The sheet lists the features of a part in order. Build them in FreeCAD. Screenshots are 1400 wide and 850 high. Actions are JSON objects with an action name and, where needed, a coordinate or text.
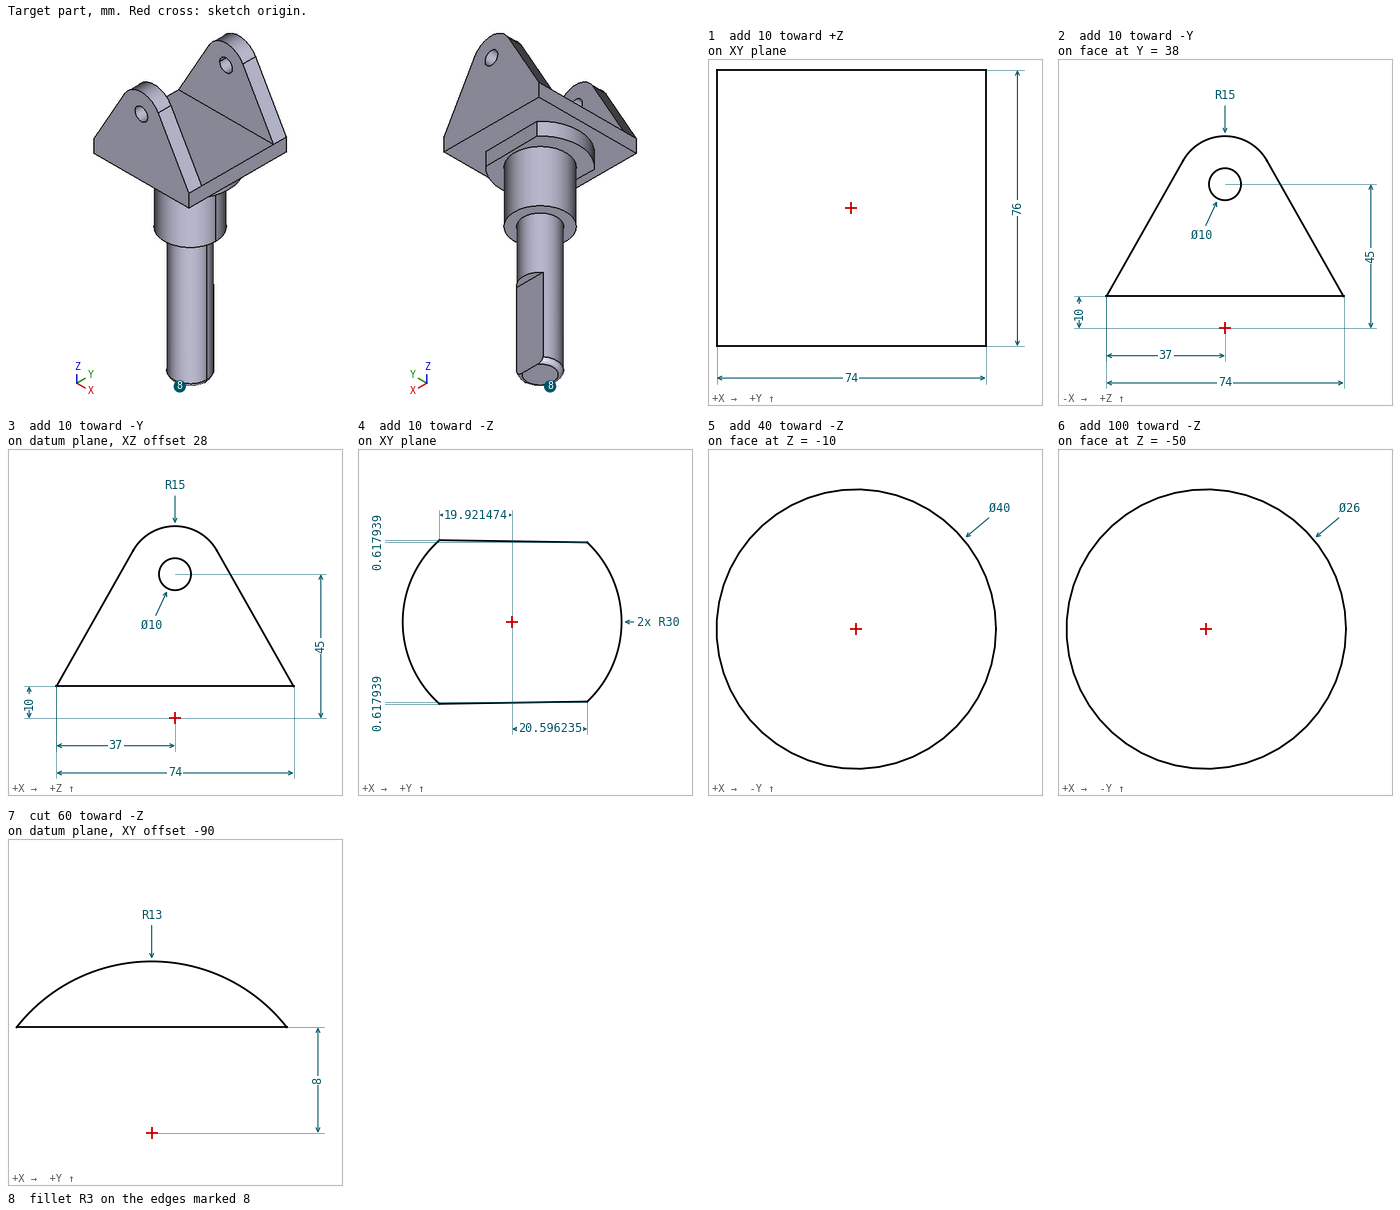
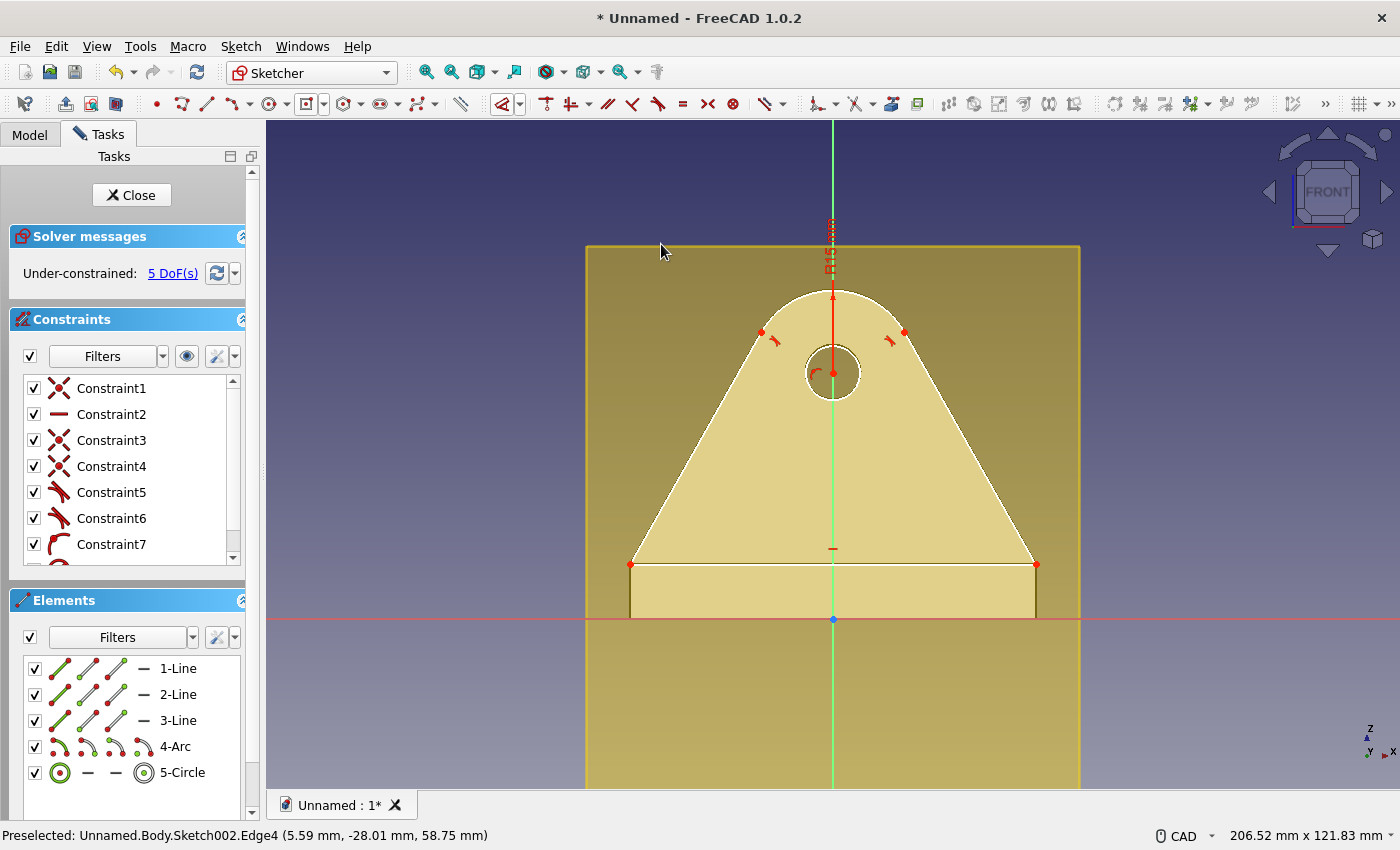
{"action": "left_click", "coordinate": [852, 354]}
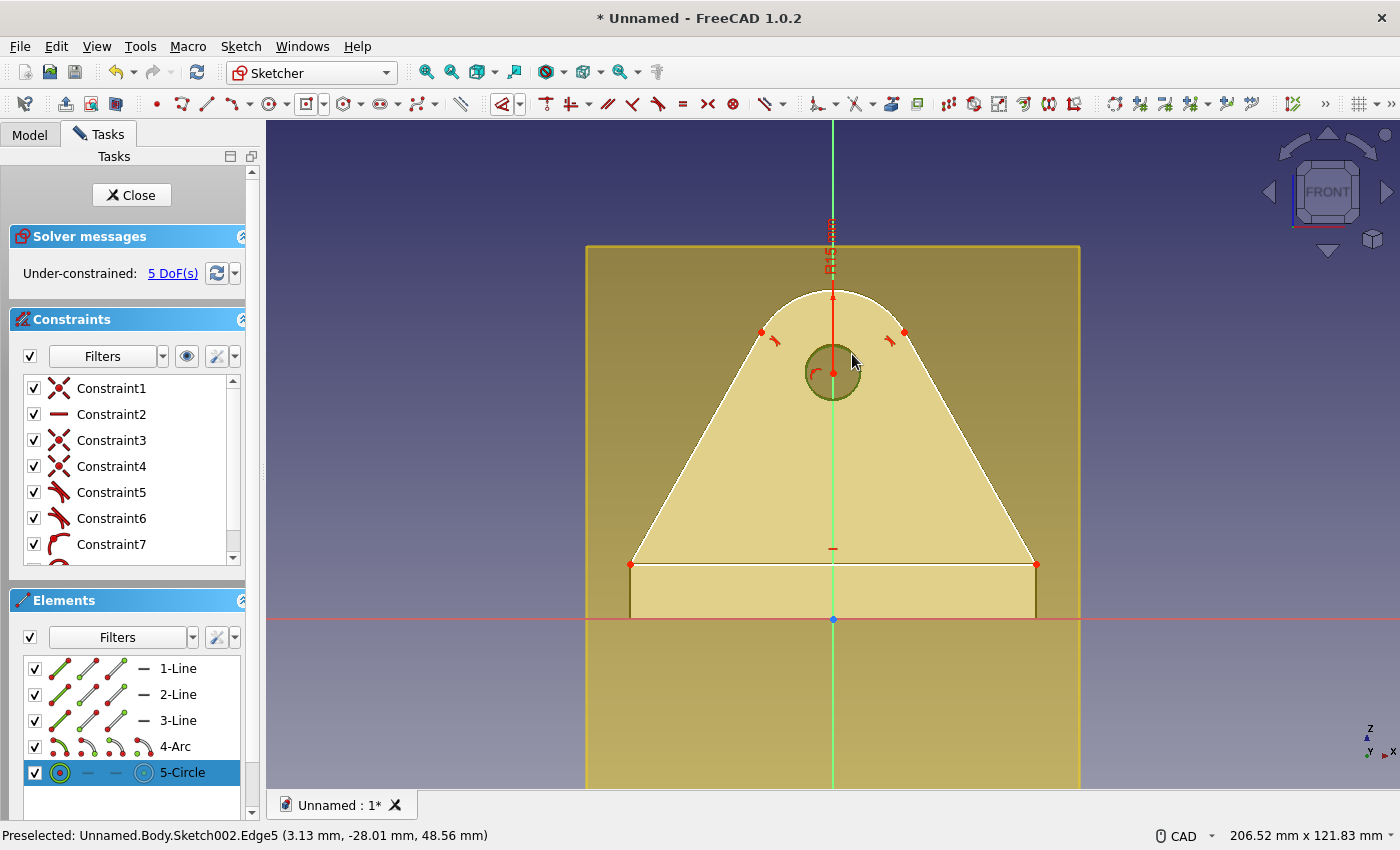
{"action": "key", "text": "k o"}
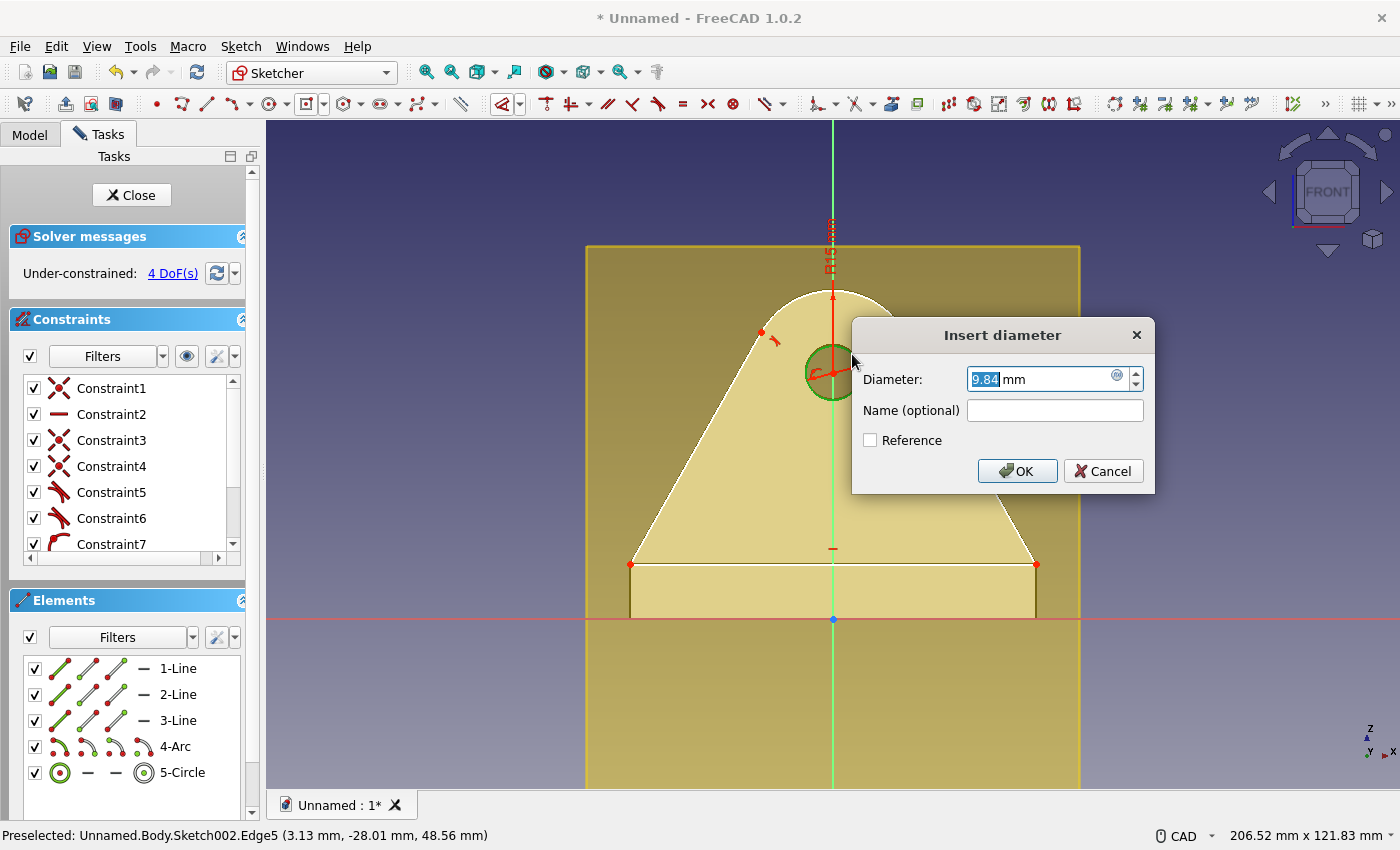
{"action": "type", "text": "10"}
{"action": "key", "text": "Return"}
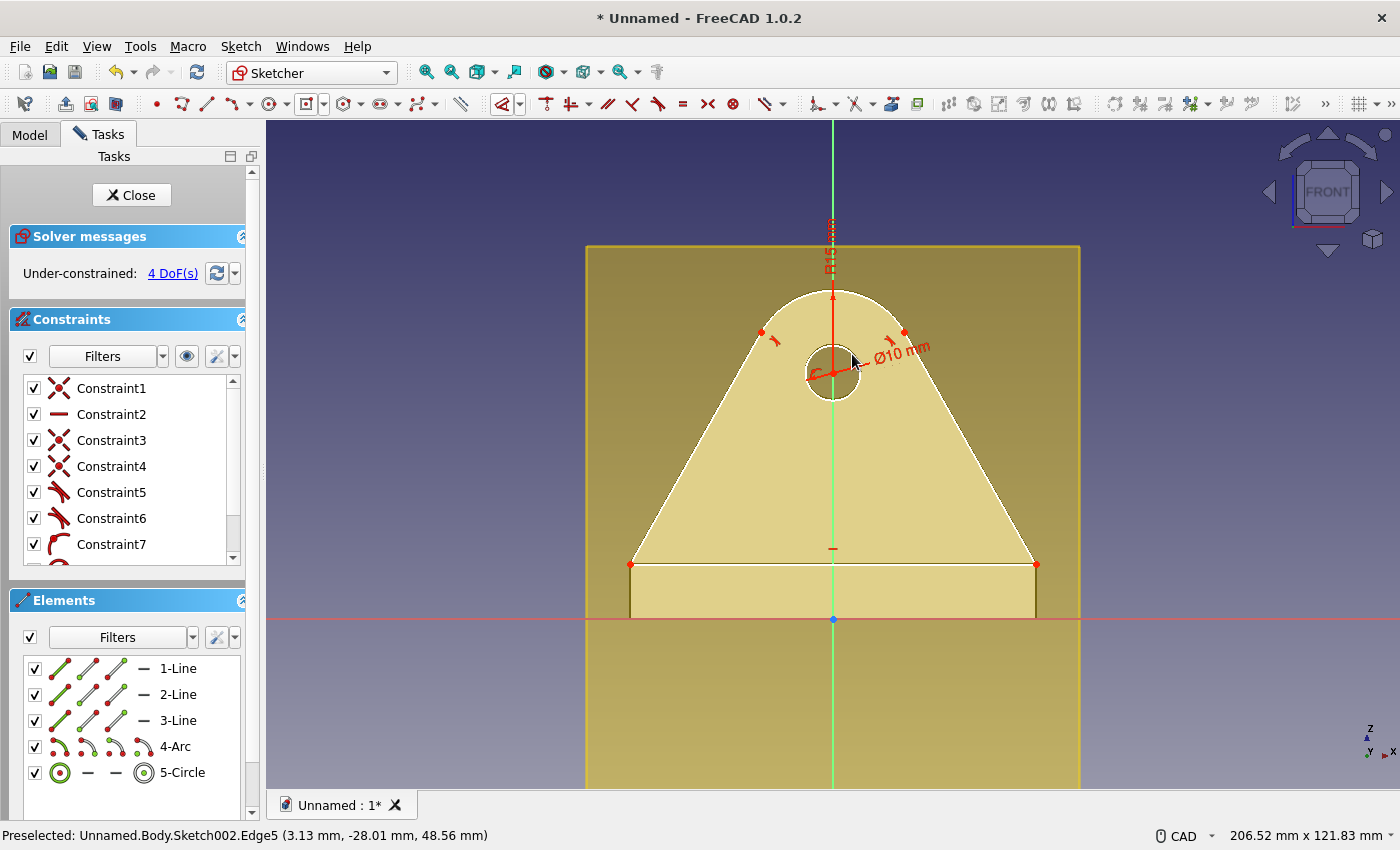
{"action": "left_click", "coordinate": [752, 565]}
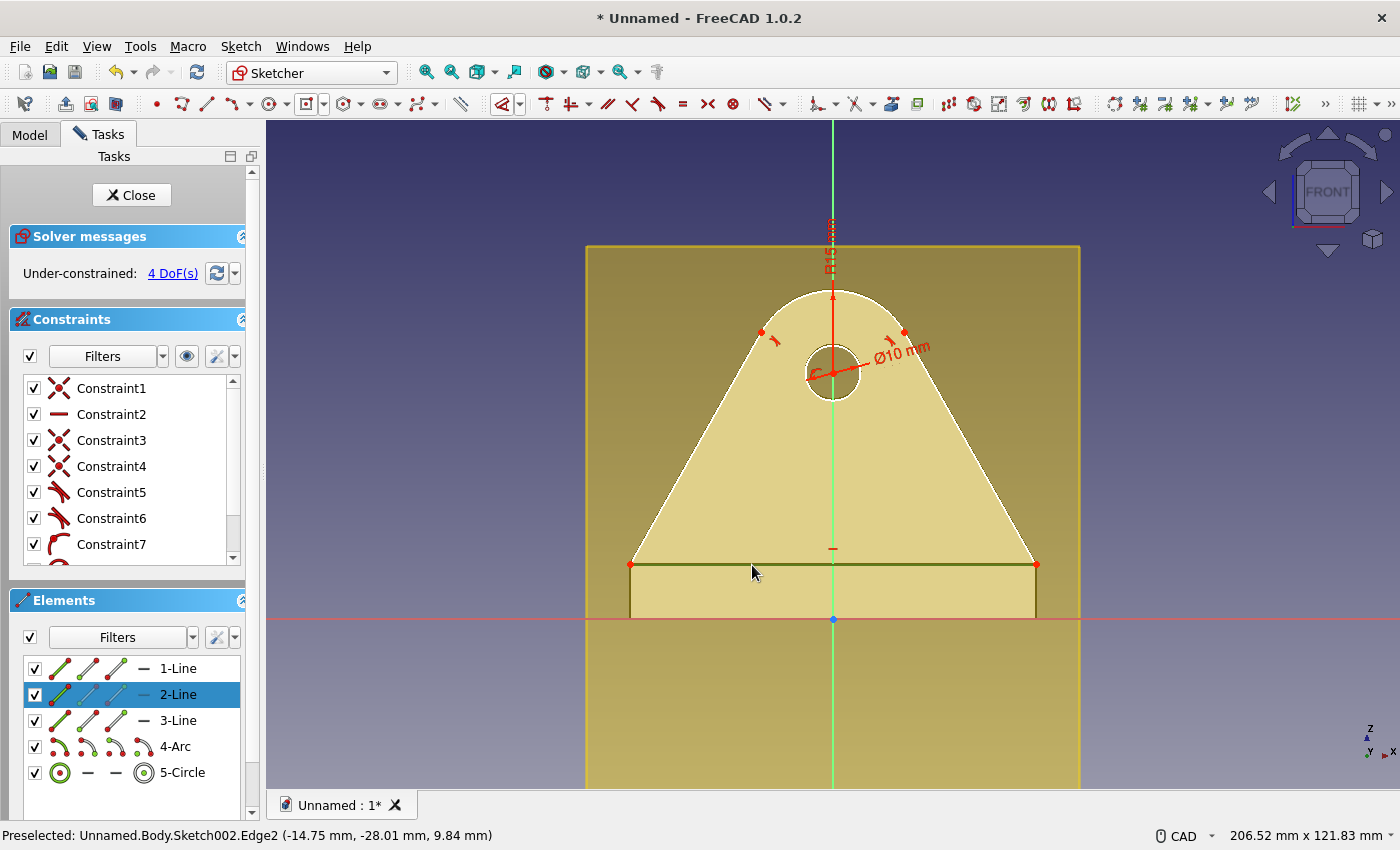
{"action": "key", "text": "l"}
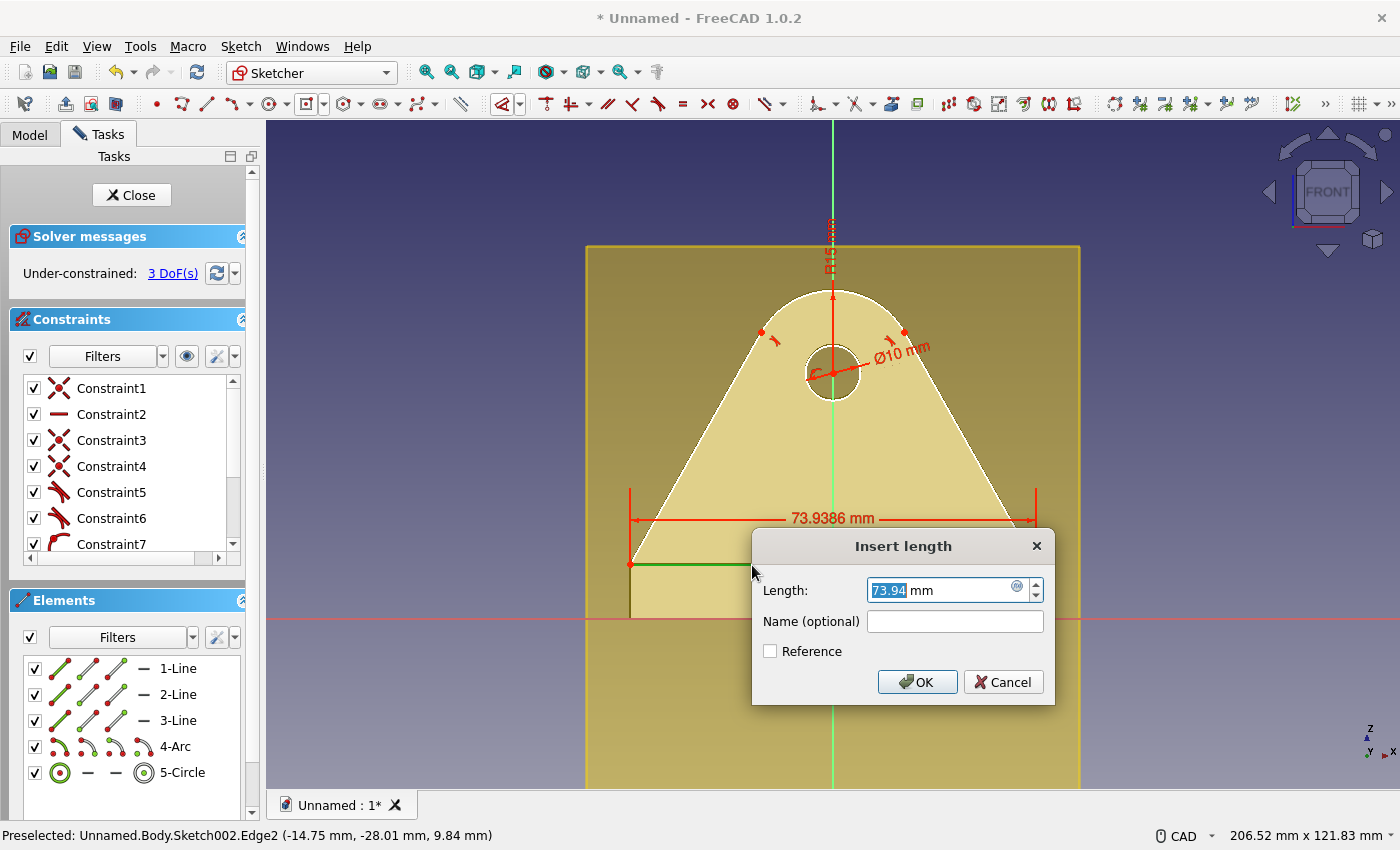
{"action": "type", "text": "74"}
{"action": "key", "text": "Return"}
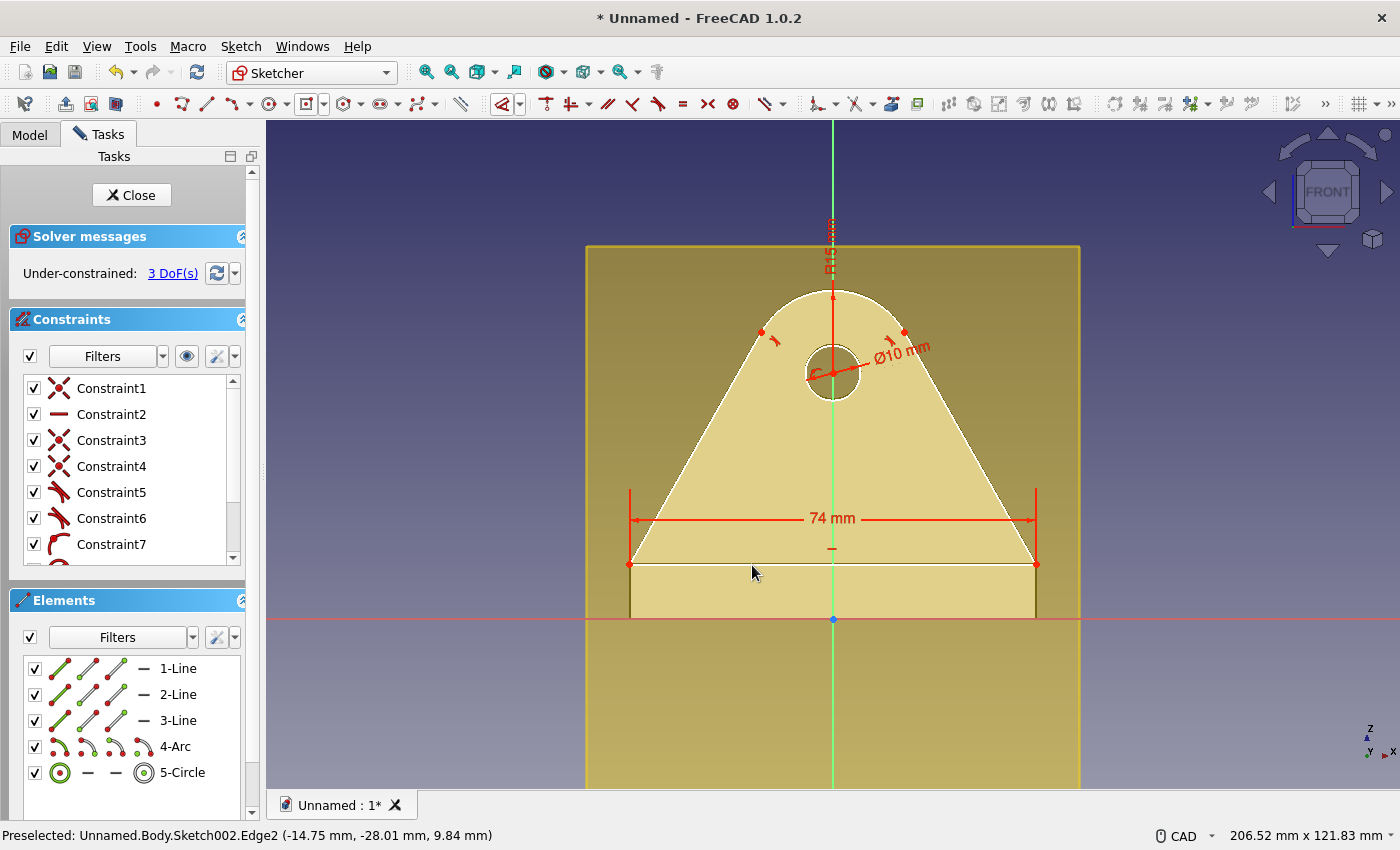
{"action": "left_click", "coordinate": [833, 373]}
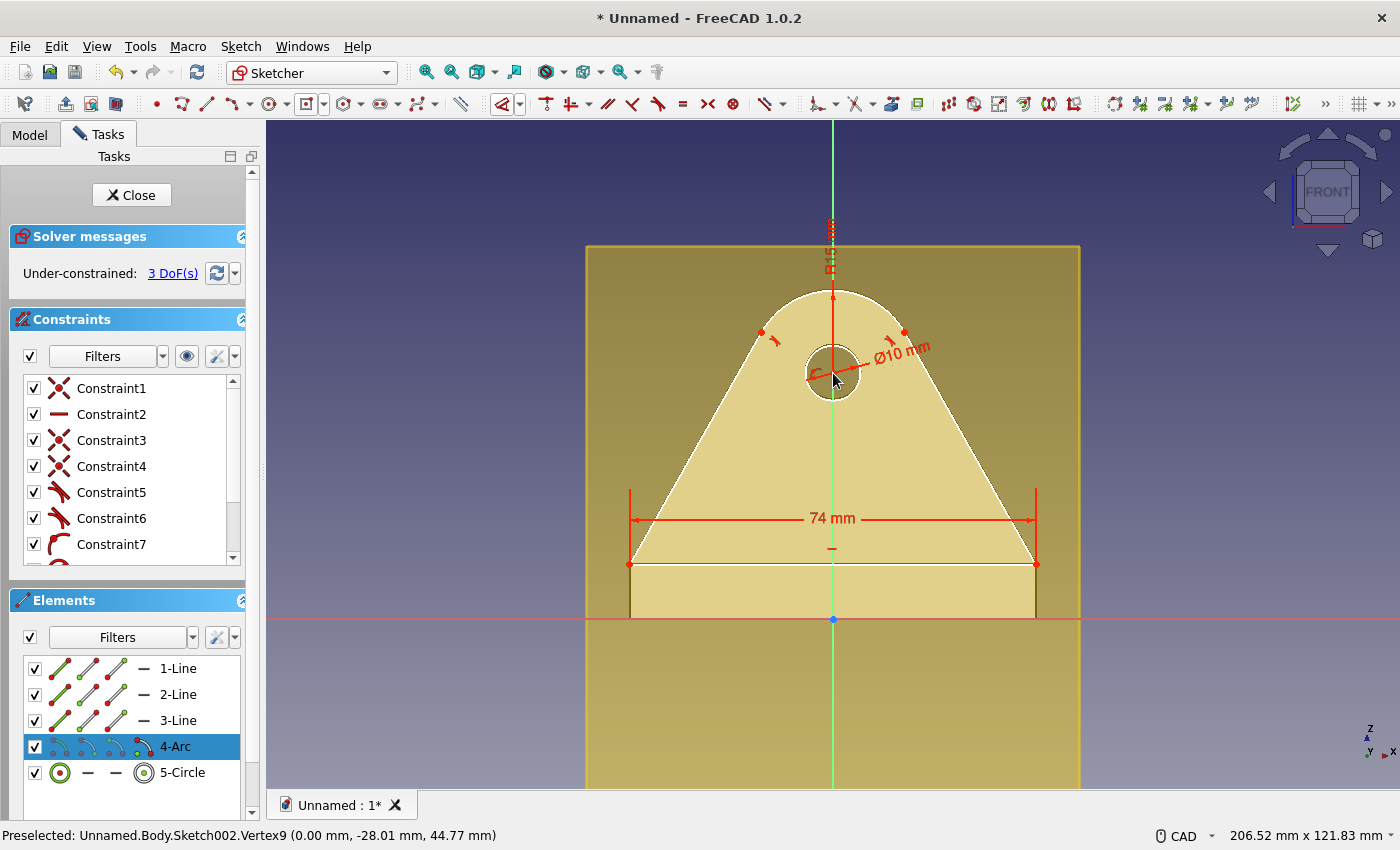
{"action": "left_click", "coordinate": [520, 104]}